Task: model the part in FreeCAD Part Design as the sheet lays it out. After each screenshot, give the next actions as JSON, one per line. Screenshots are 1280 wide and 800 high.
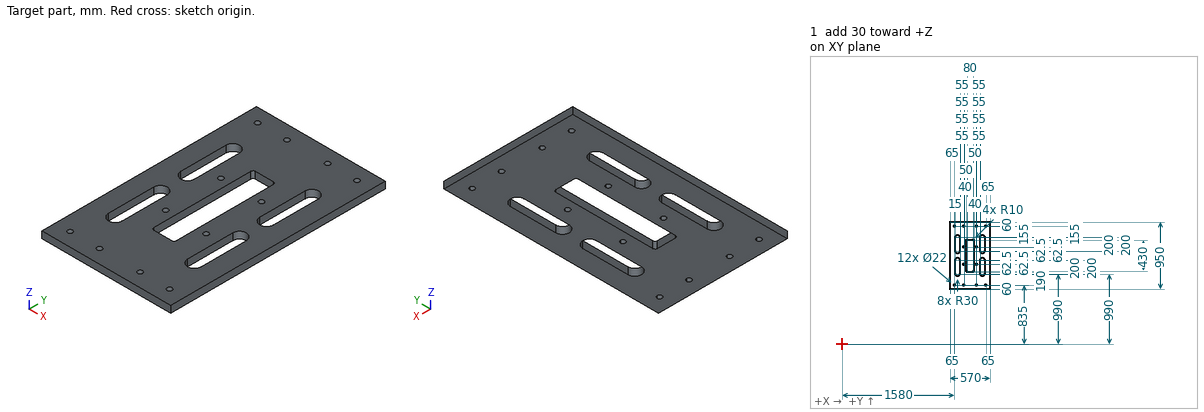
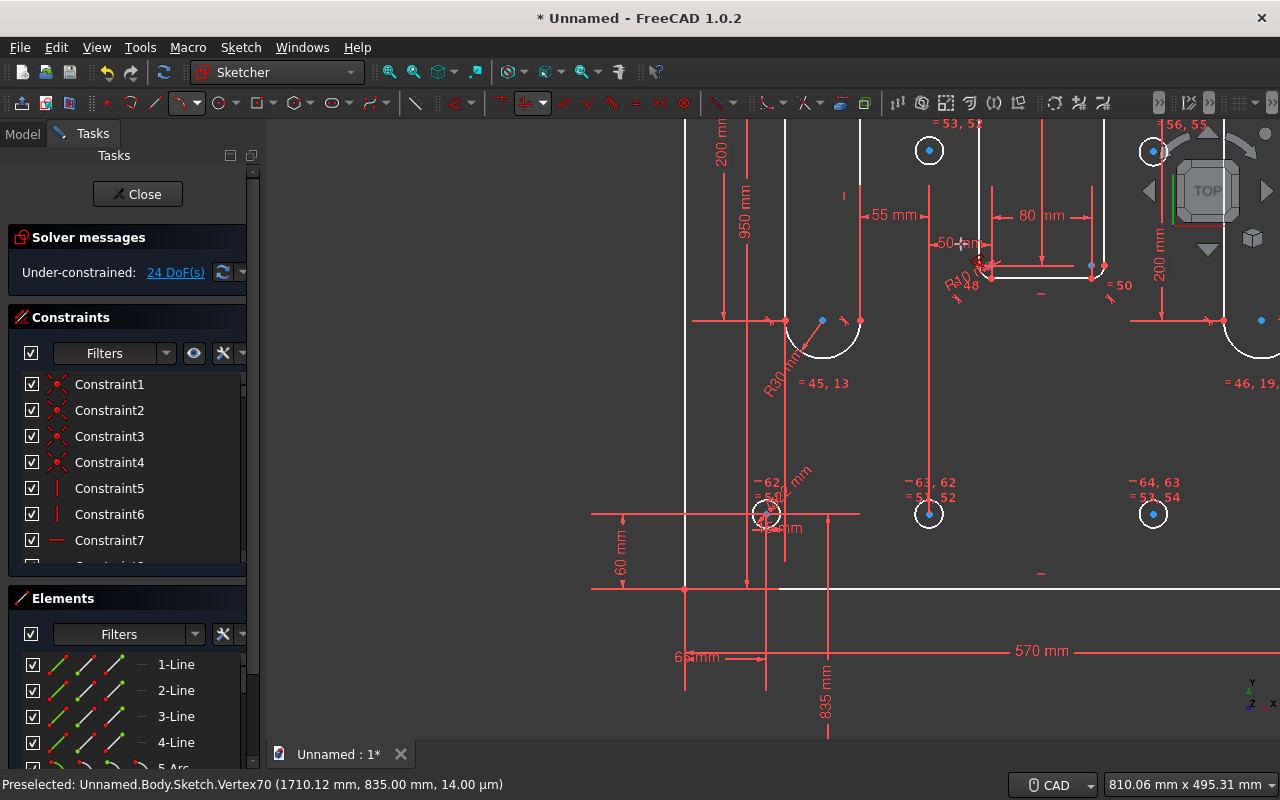
{"action": "scroll", "coordinate": [859, 416], "scroll_direction": "down", "scroll_amount": 8}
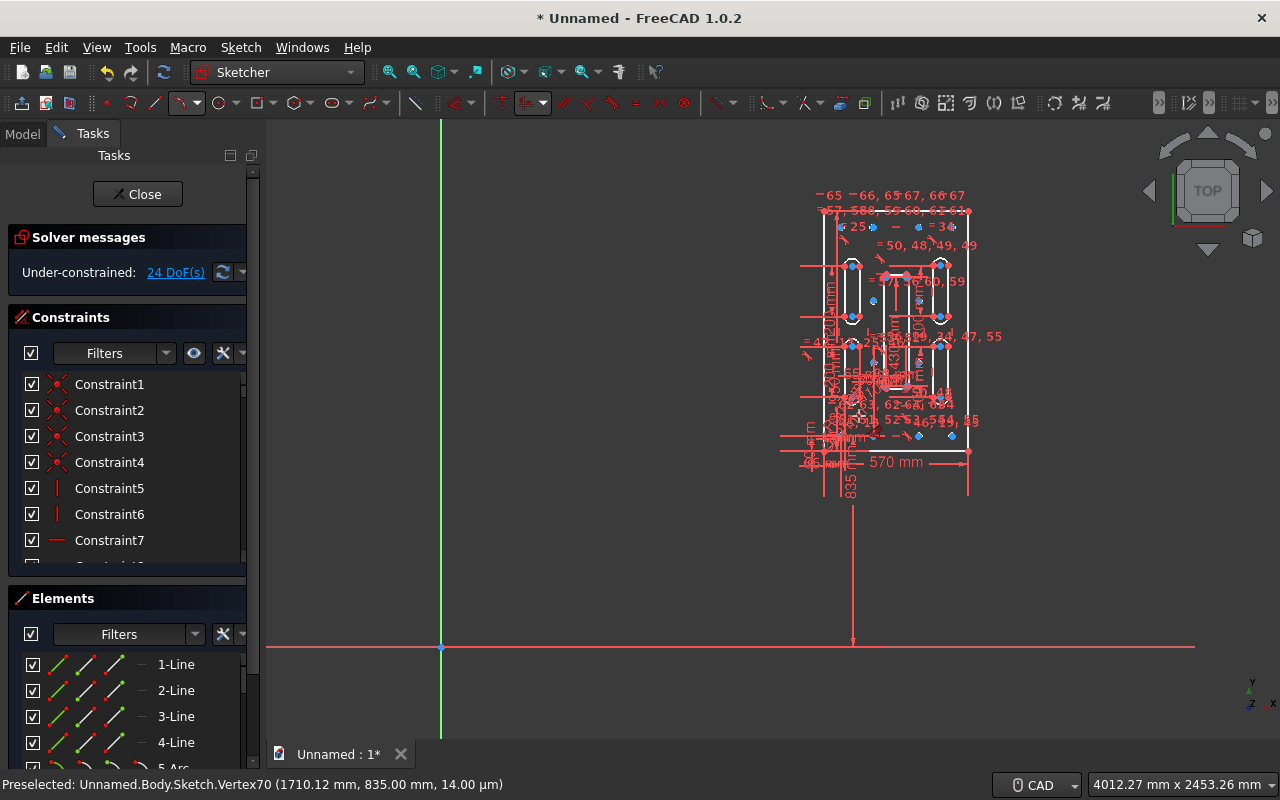
{"action": "scroll", "coordinate": [860, 347], "scroll_direction": "up", "scroll_amount": 6}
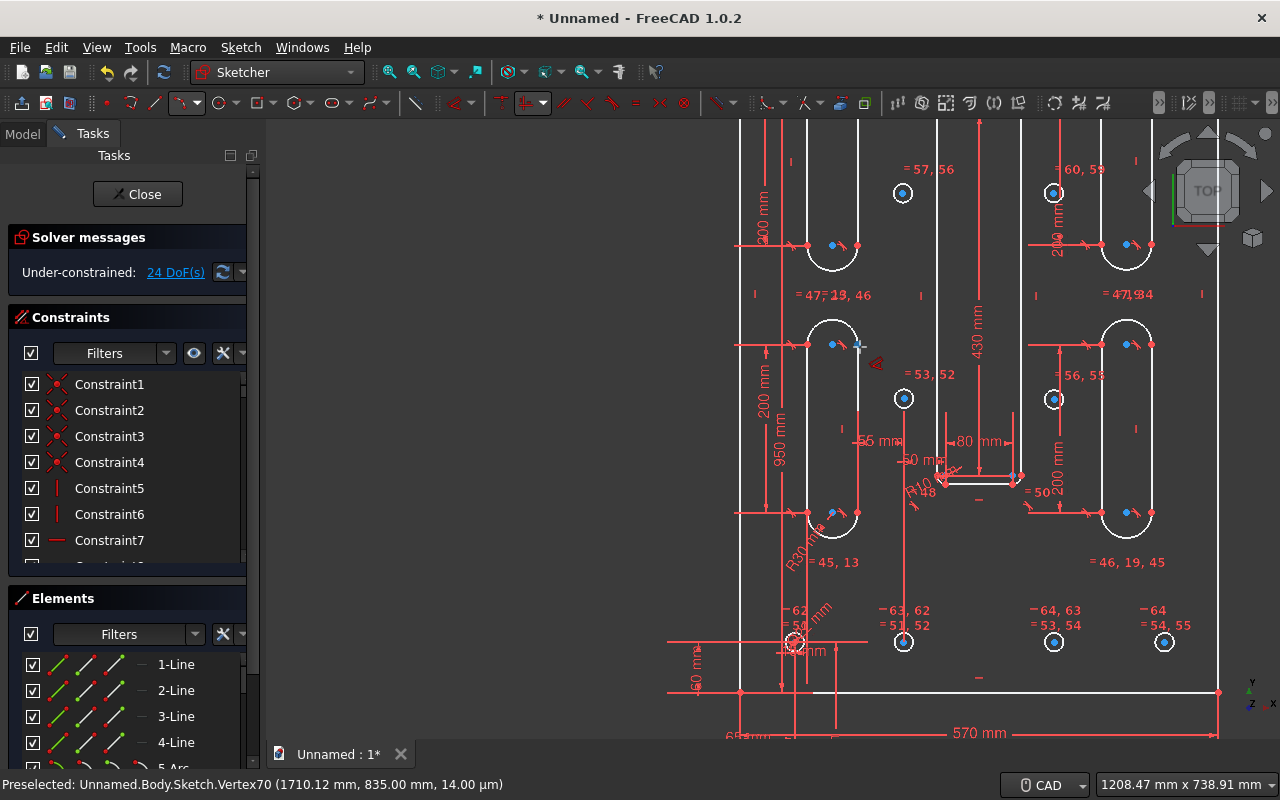
{"action": "left_click", "coordinate": [858, 345]}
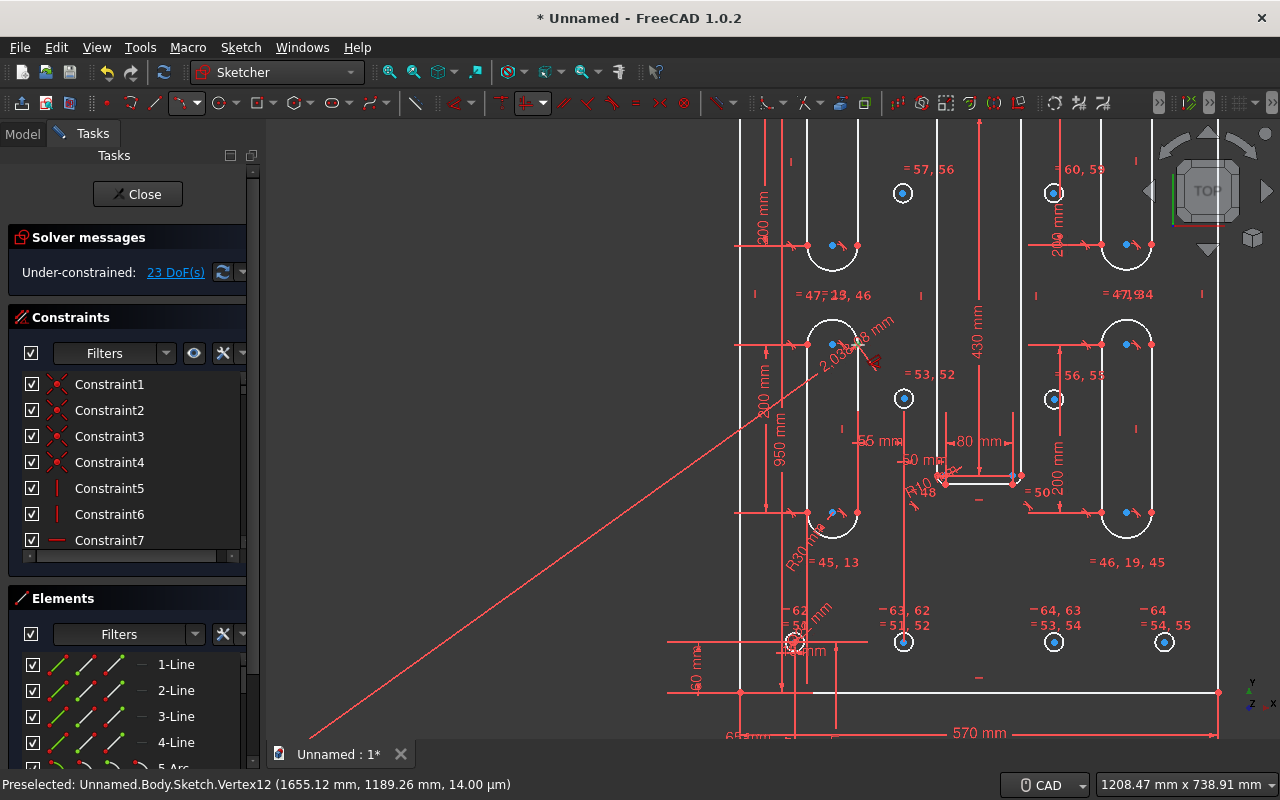
{"action": "left_click", "coordinate": [904, 399]}
{"action": "left_click", "coordinate": [881, 311]}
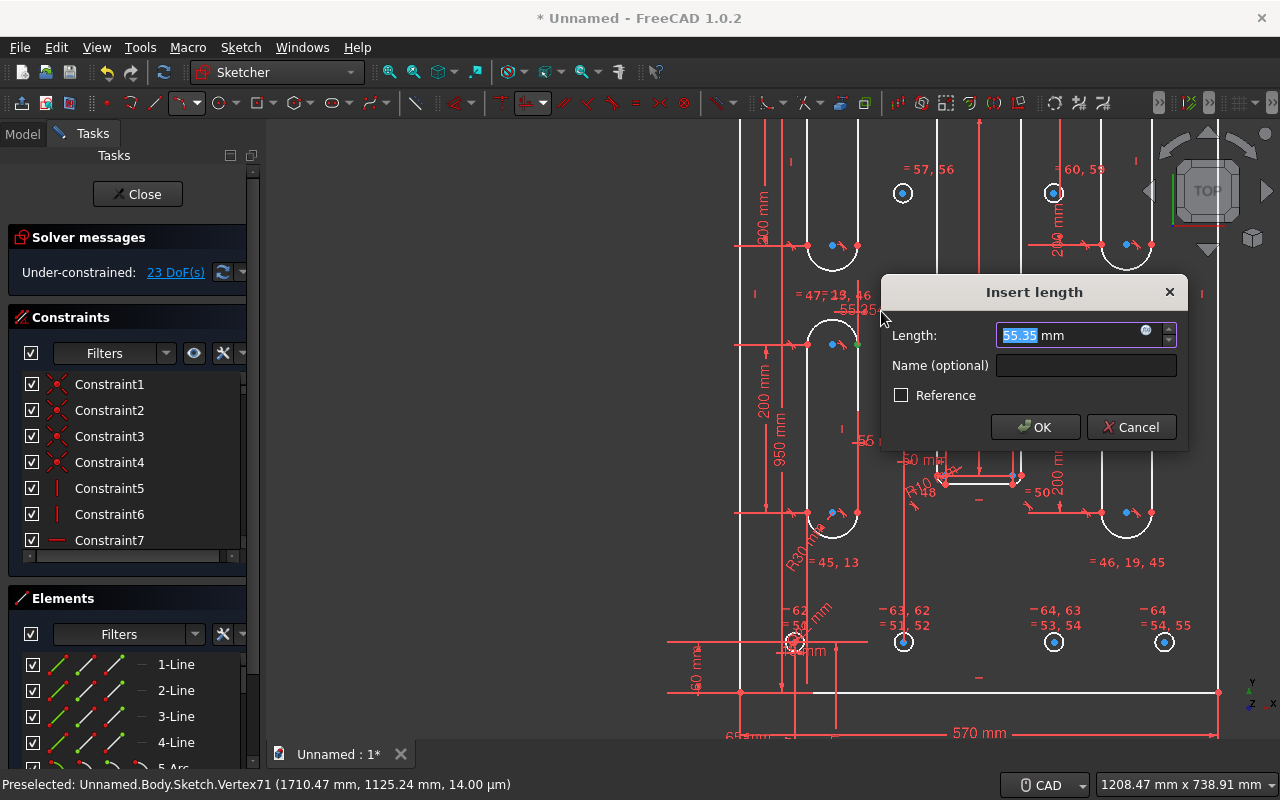
{"action": "type", "text": "55"}
{"action": "key", "text": "Return"}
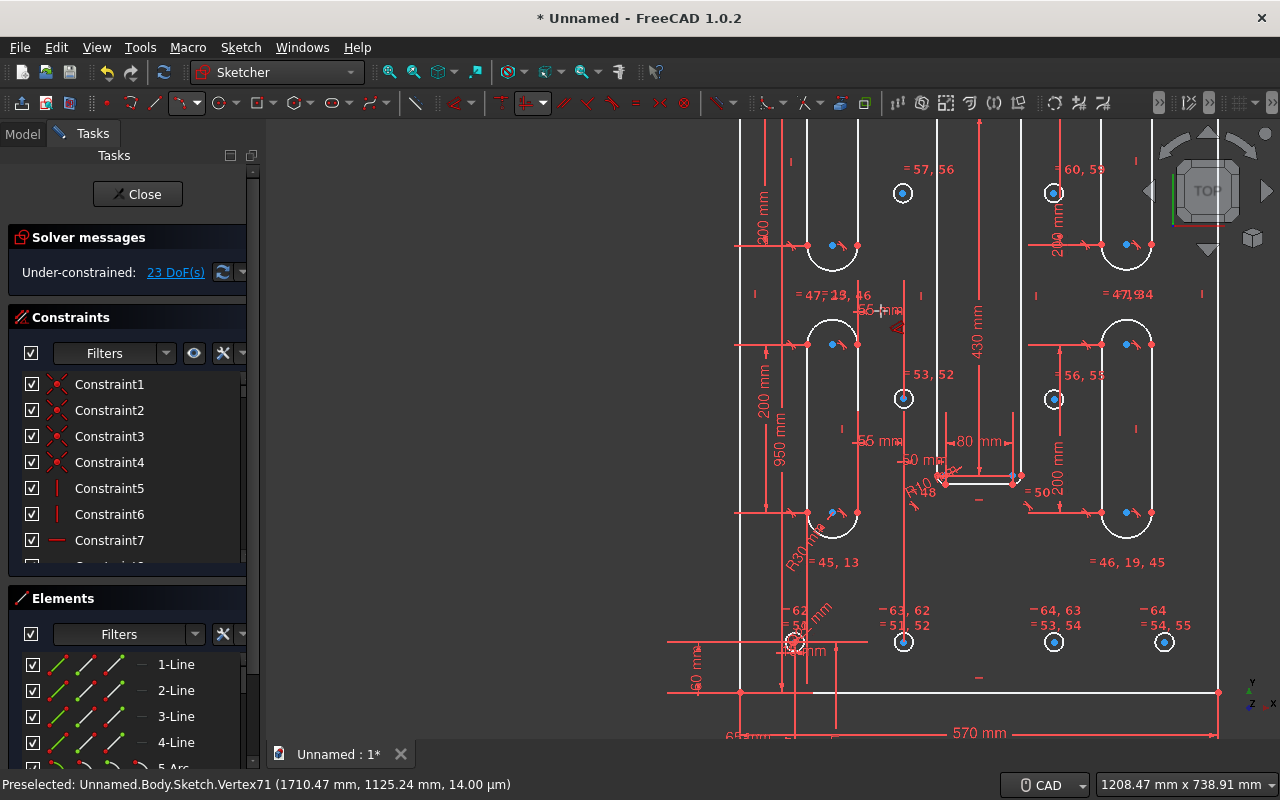
{"action": "left_click", "coordinate": [1102, 513]}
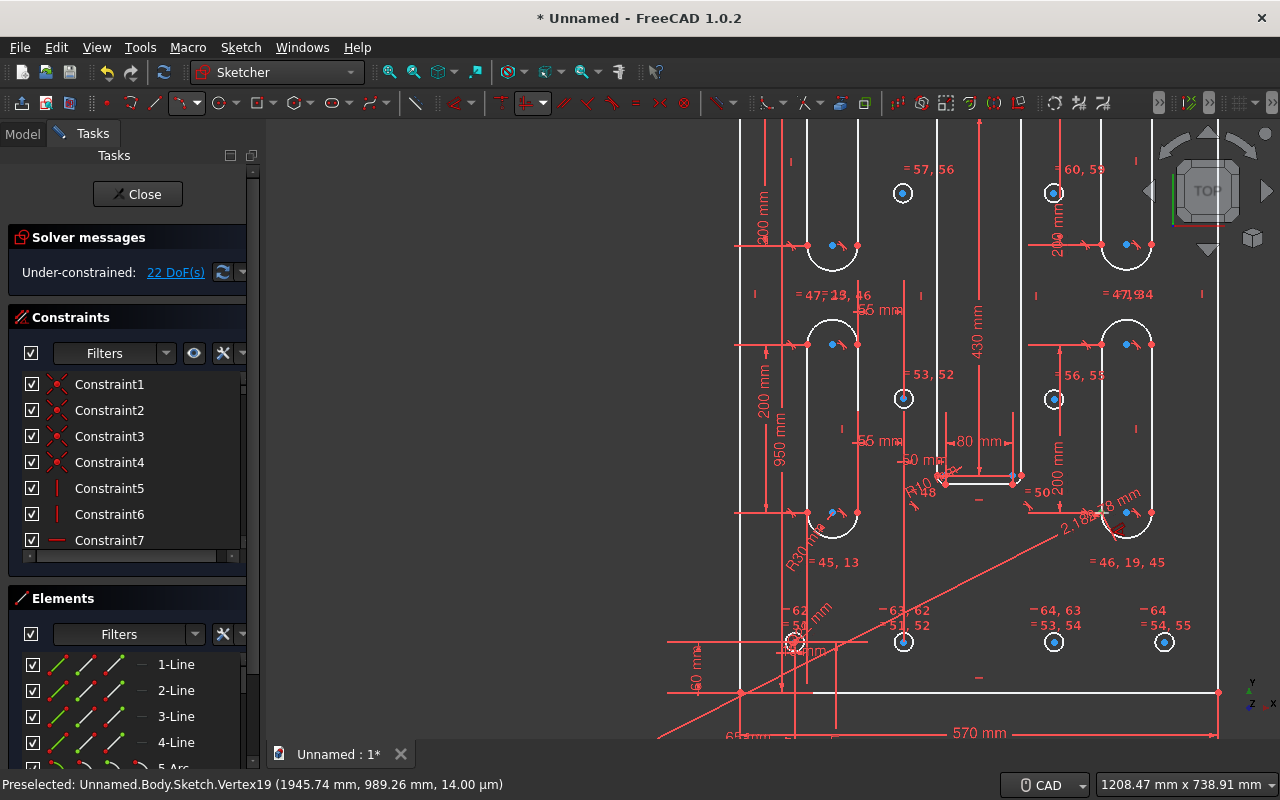
{"action": "left_click", "coordinate": [1054, 642]}
{"action": "left_click", "coordinate": [1078, 676]}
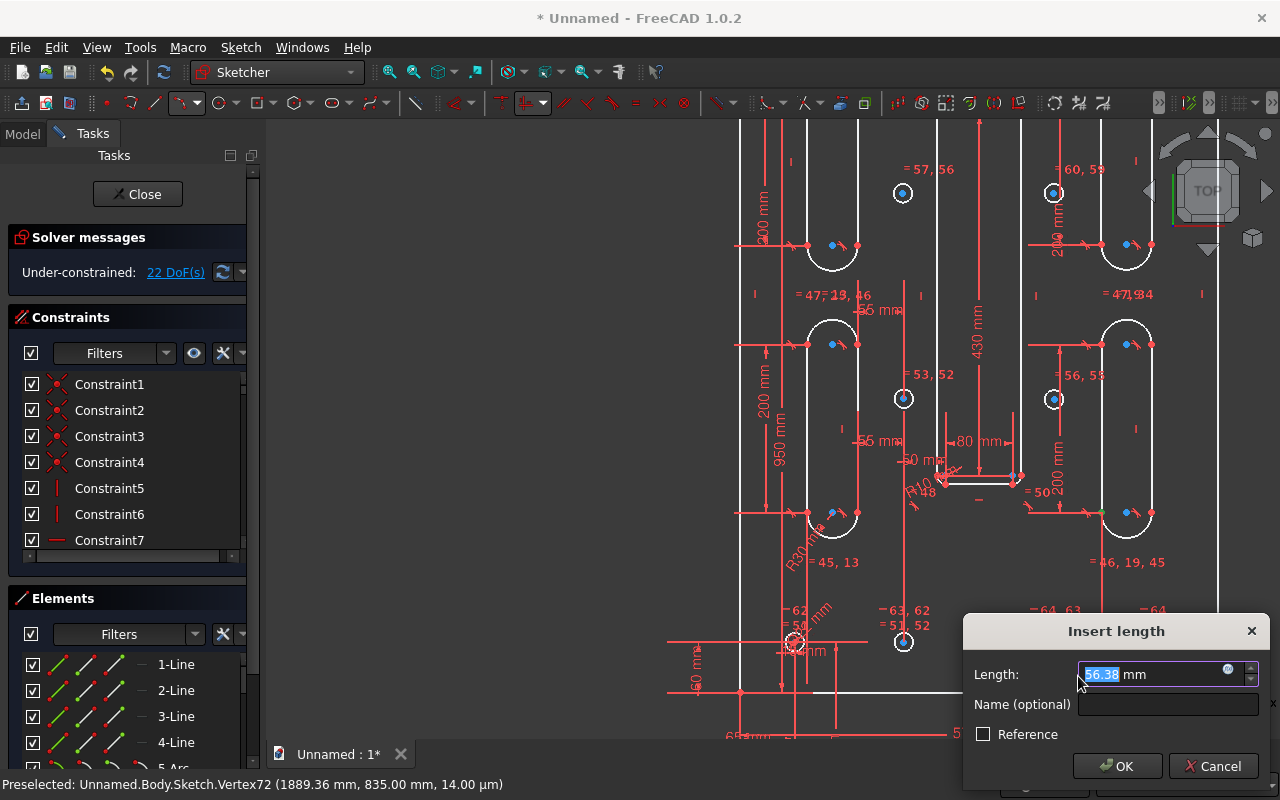
{"action": "type", "text": "55"}
{"action": "key", "text": "Return"}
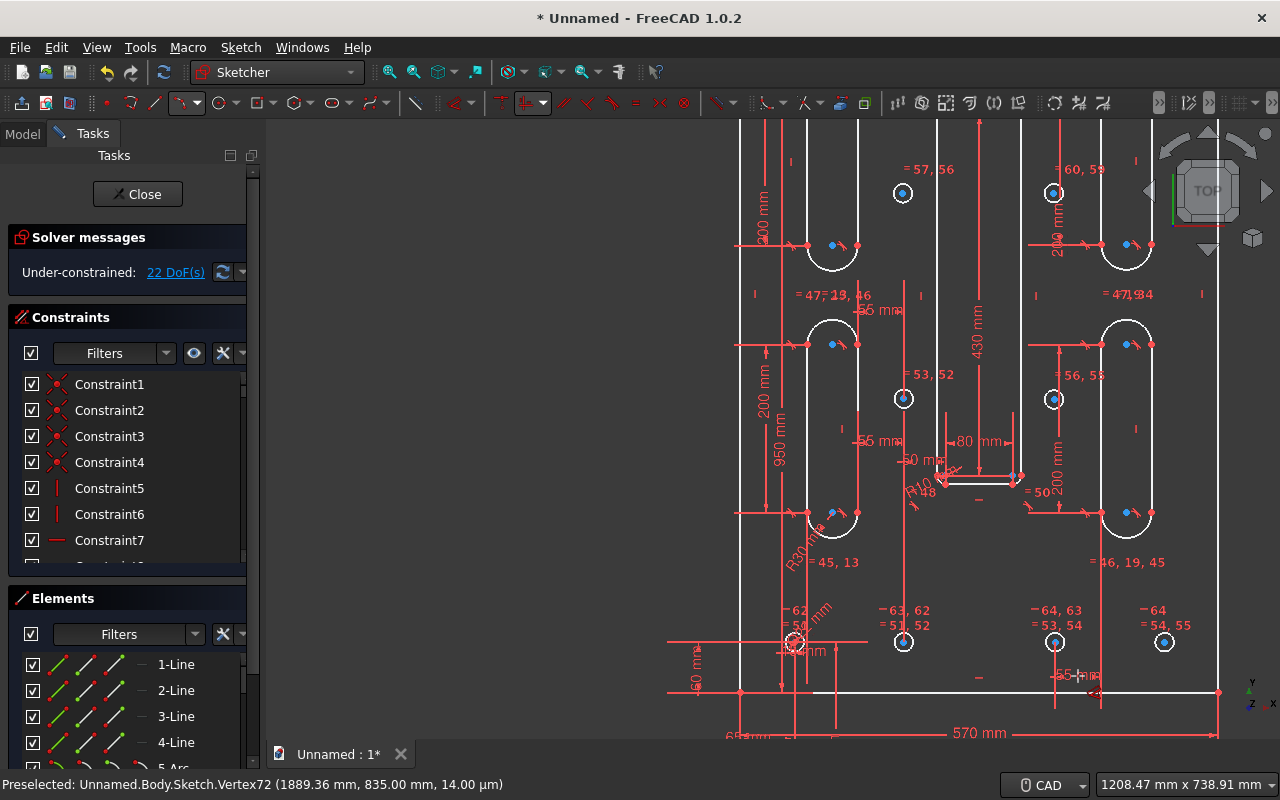
{"action": "scroll", "coordinate": [1013, 484], "scroll_direction": "up", "scroll_amount": 2}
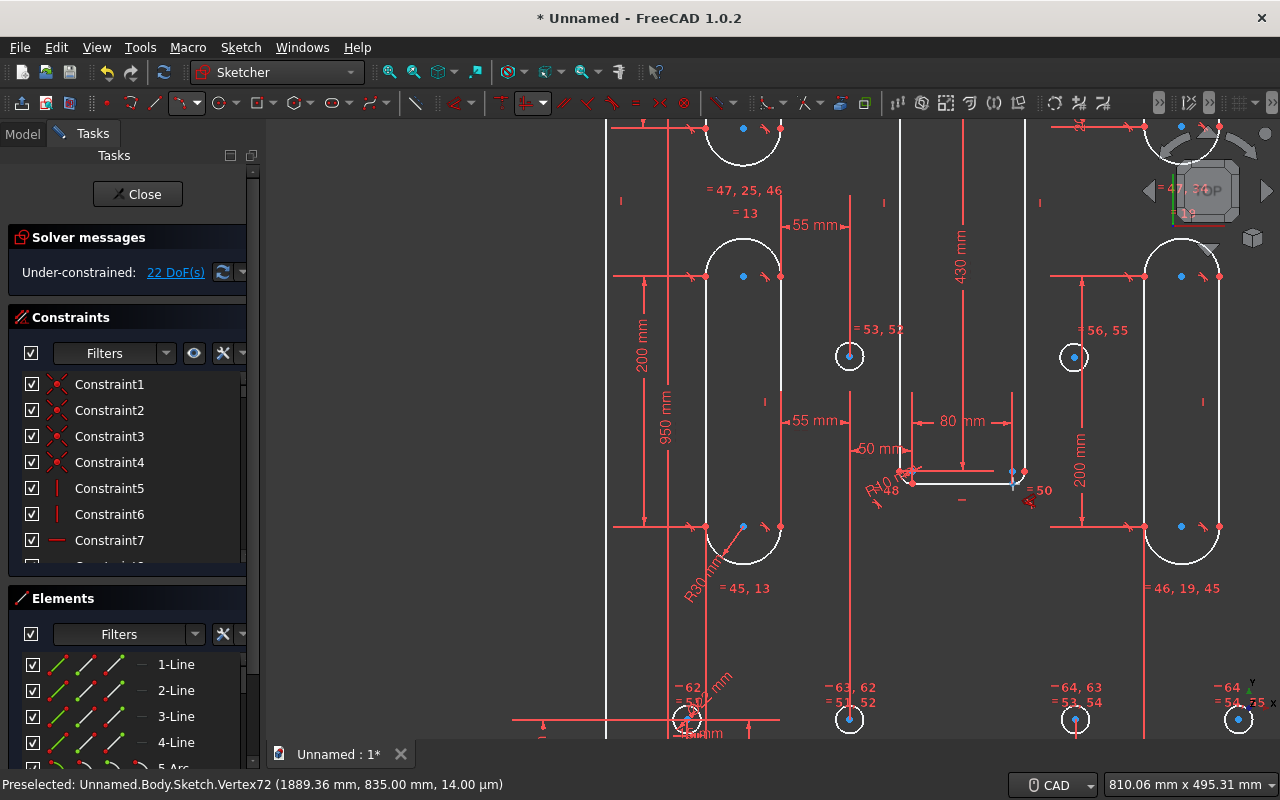
{"action": "left_click", "coordinate": [1012, 484]}